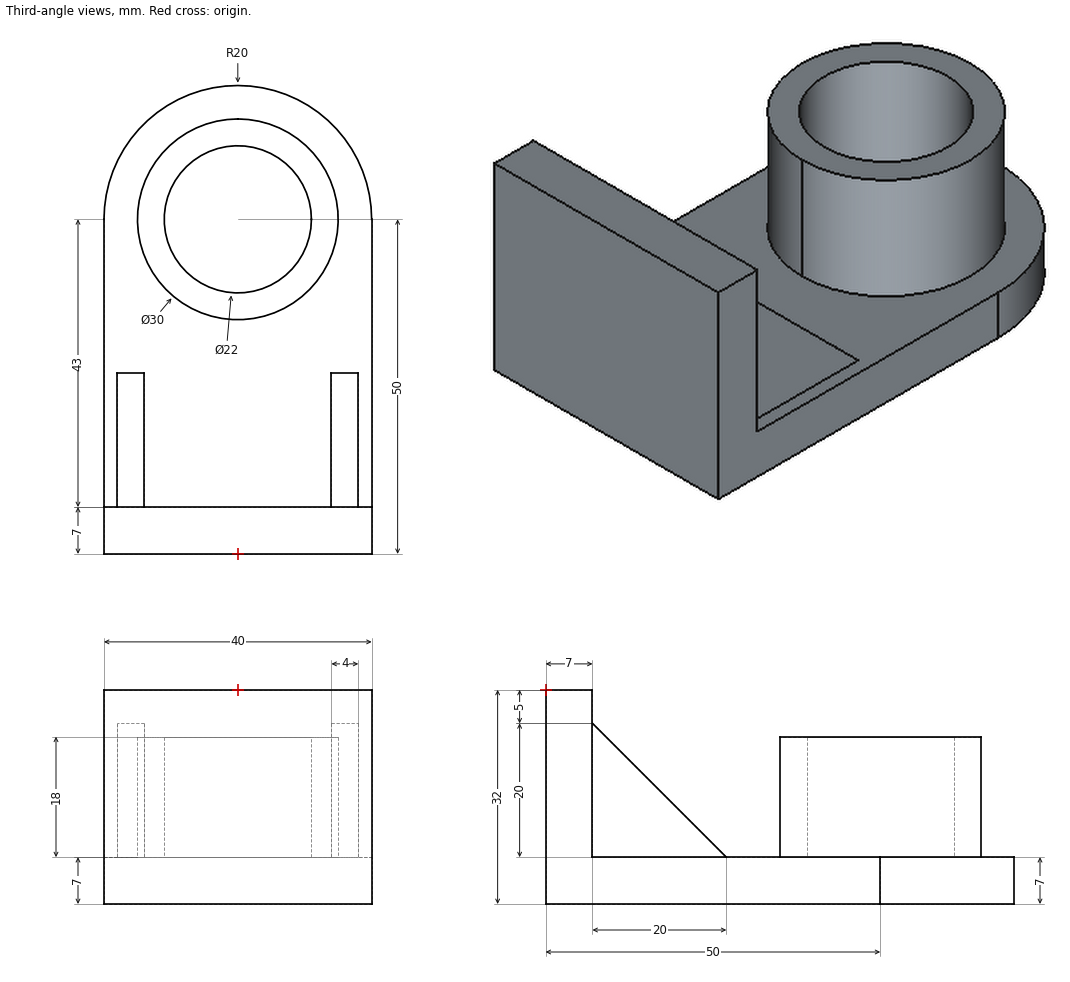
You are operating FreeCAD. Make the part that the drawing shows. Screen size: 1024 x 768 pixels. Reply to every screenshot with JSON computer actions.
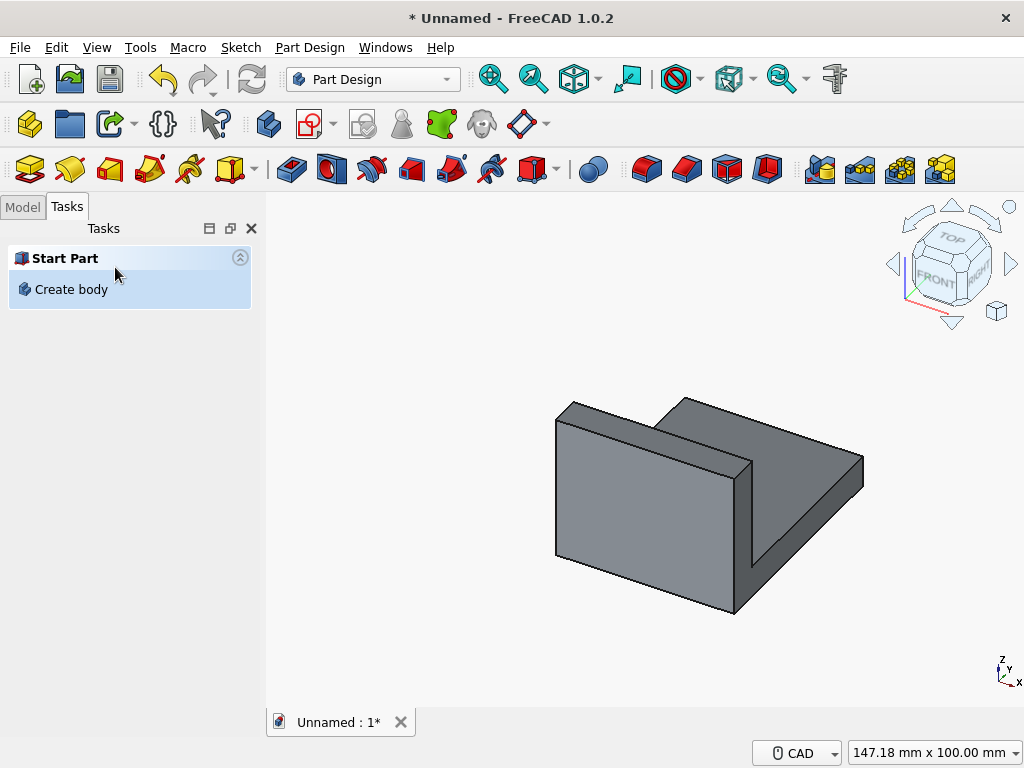
{"action": "key", "text": "0"}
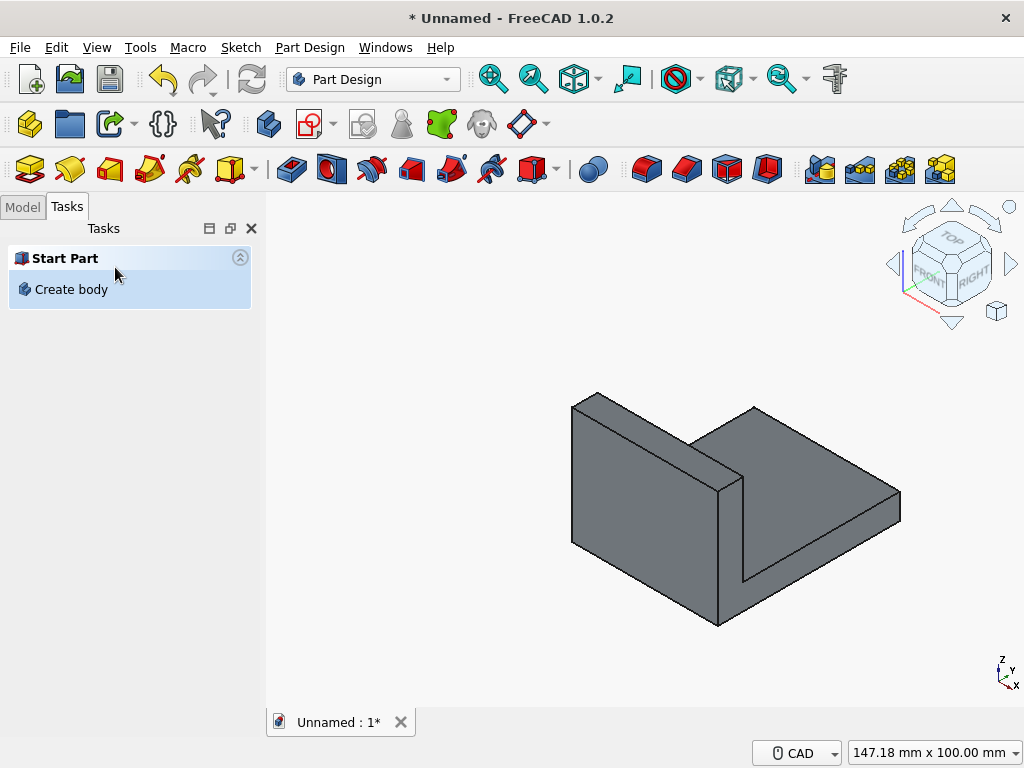
{"action": "left_click", "coordinate": [771, 481]}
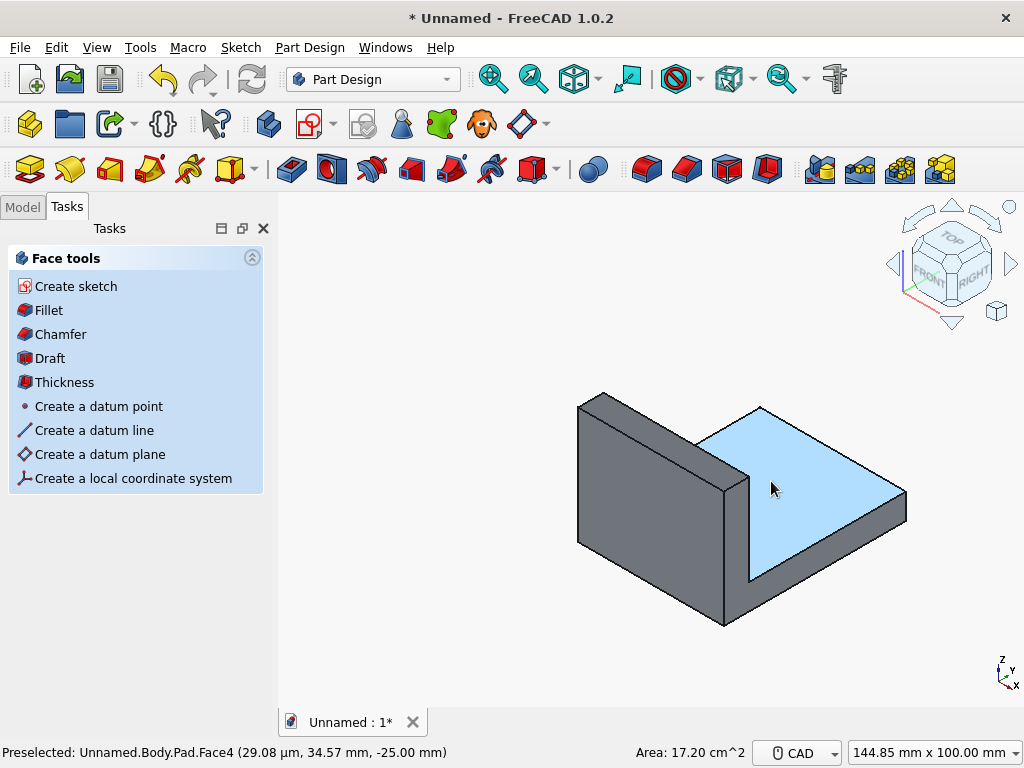
{"action": "left_click", "coordinate": [310, 124]}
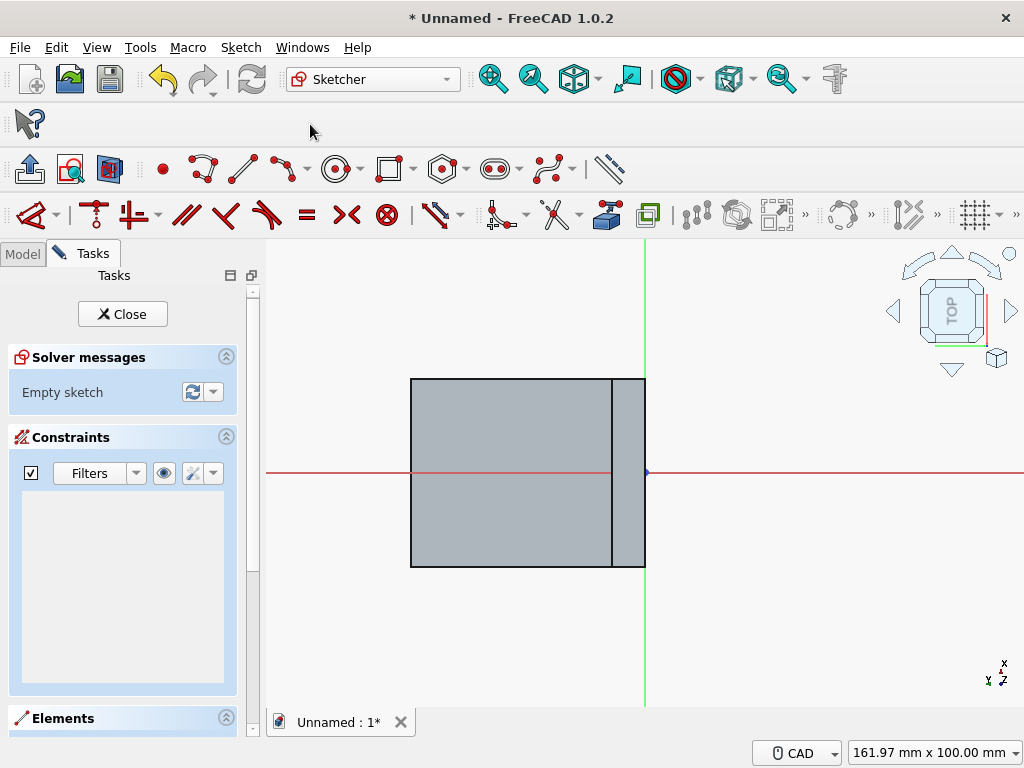
{"action": "scroll", "coordinate": [294, 473], "scroll_direction": "up", "scroll_amount": 1}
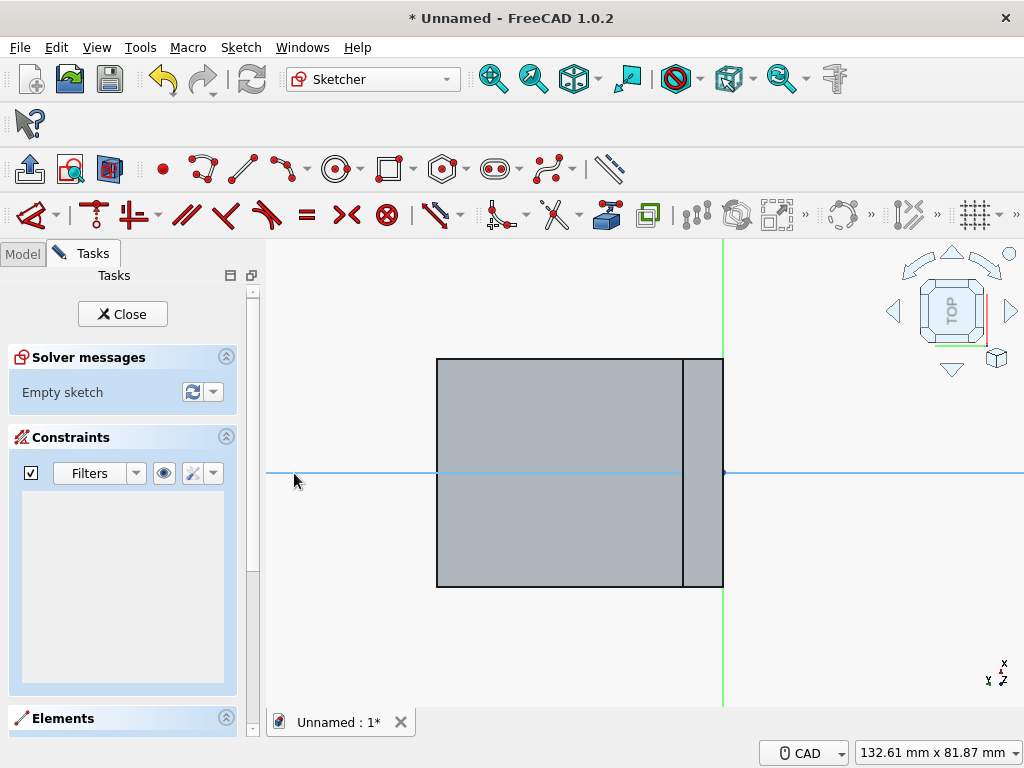
{"action": "key", "text": "g m"}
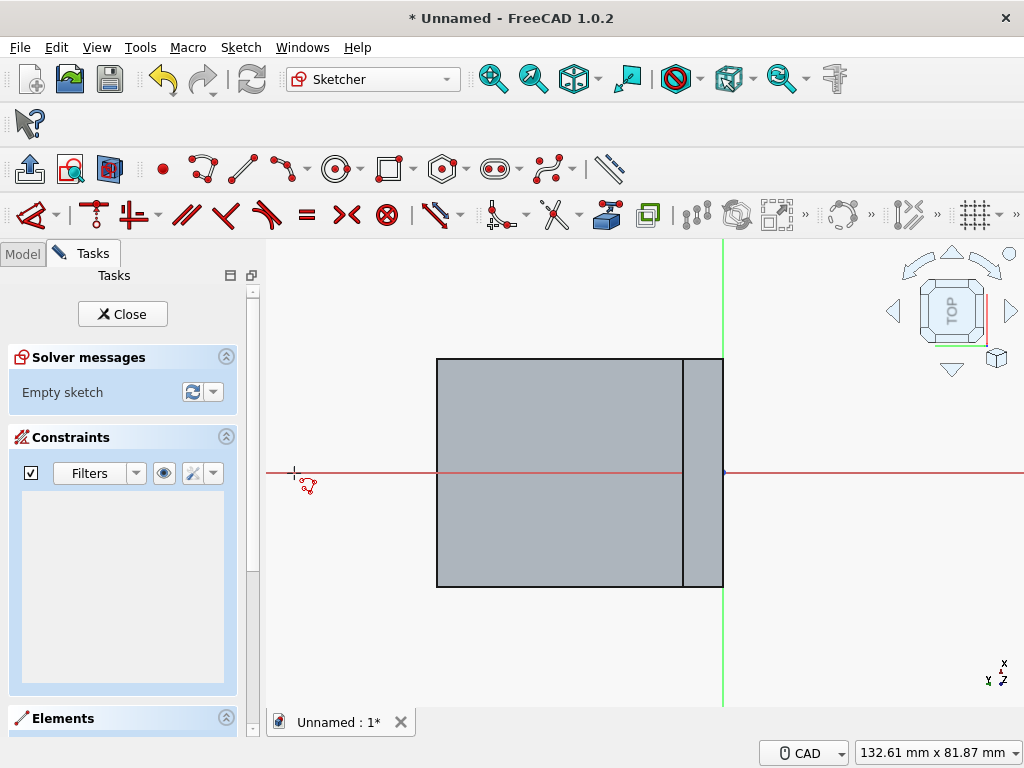
{"action": "left_click", "coordinate": [437, 587]}
{"action": "left_click", "coordinate": [683, 587]}
{"action": "left_click", "coordinate": [683, 359]}
{"action": "left_click", "coordinate": [437, 359]}
{"action": "right_click", "coordinate": [437, 359]}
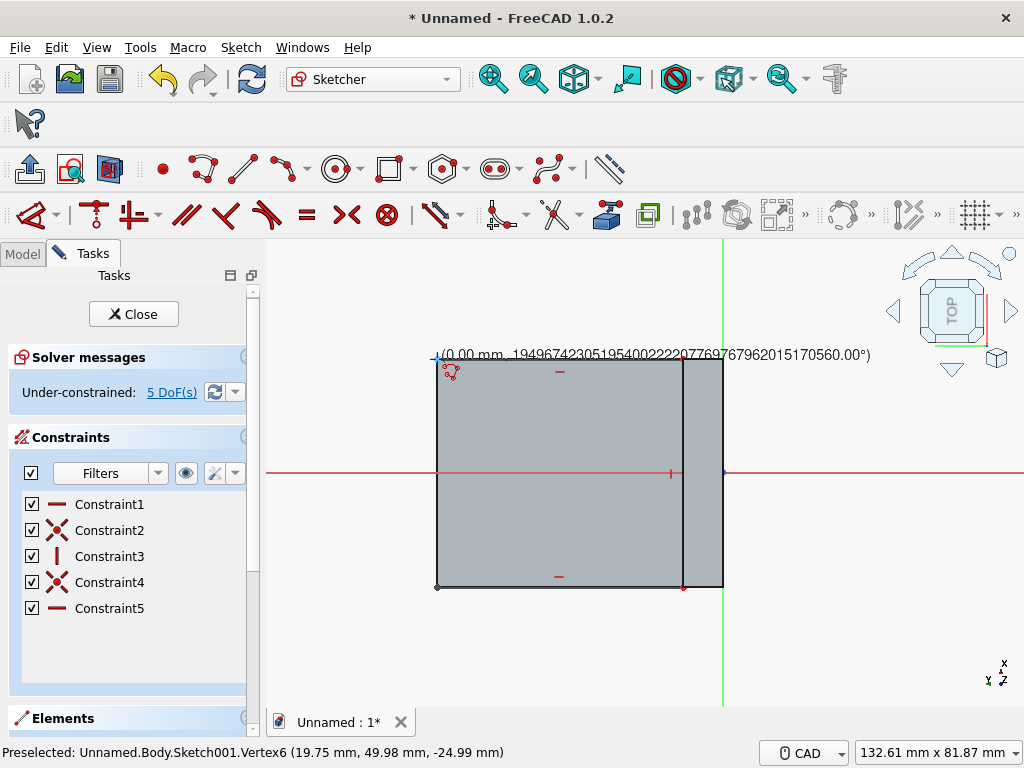
{"action": "left_click", "coordinate": [284, 170]}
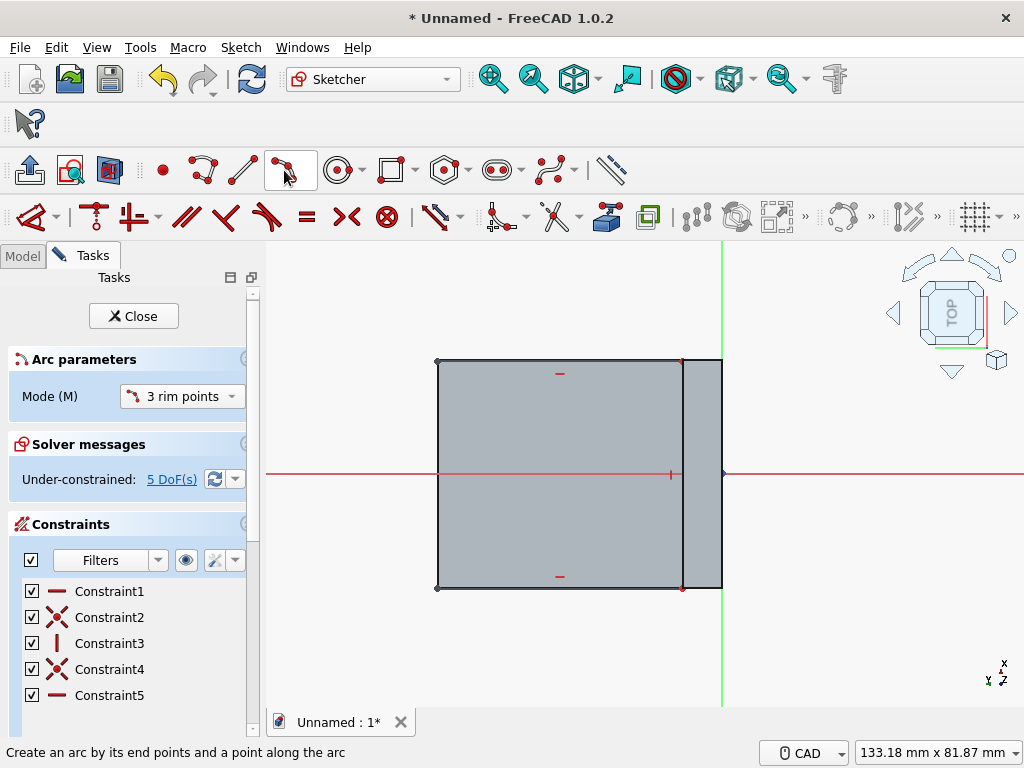
{"action": "left_click", "coordinate": [438, 361]}
{"action": "left_click", "coordinate": [438, 589]}
{"action": "left_click", "coordinate": [330, 439]}
{"action": "key", "text": "Escape"}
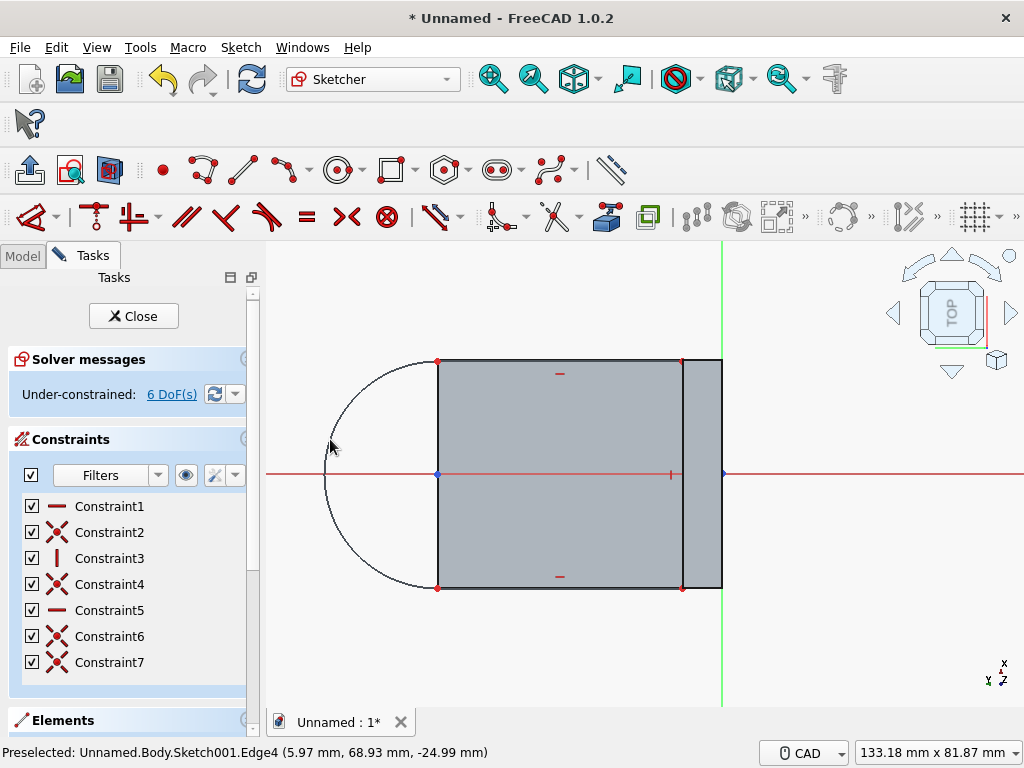
{"action": "left_click", "coordinate": [511, 589]}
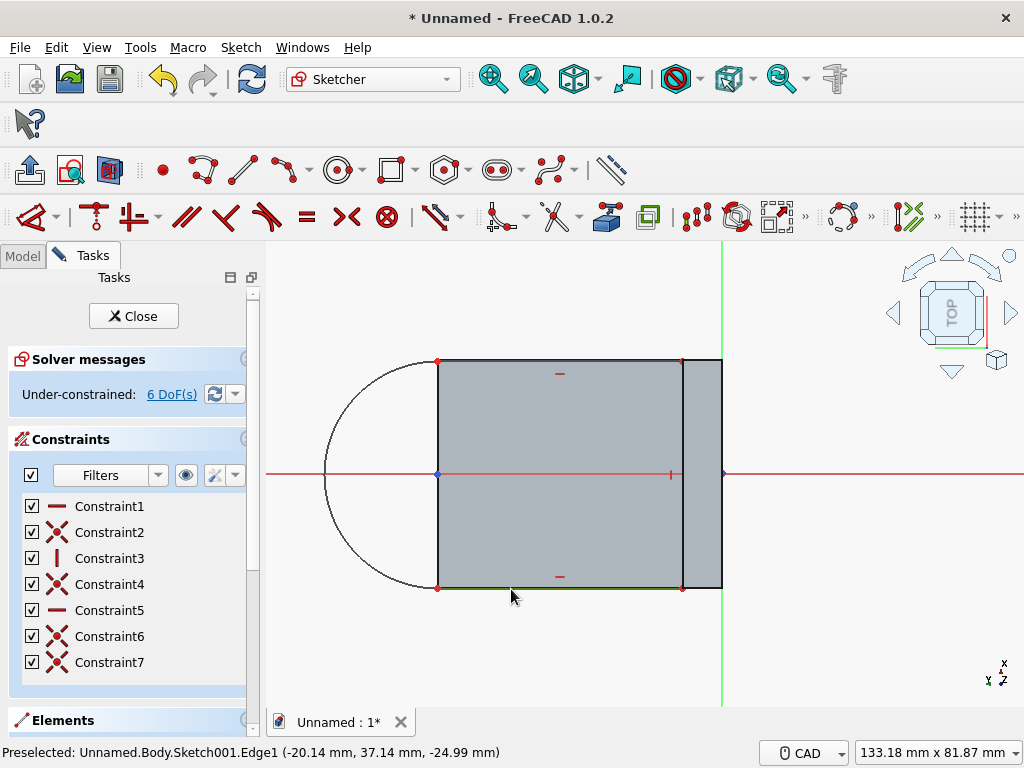
{"action": "left_click", "coordinate": [346, 408]}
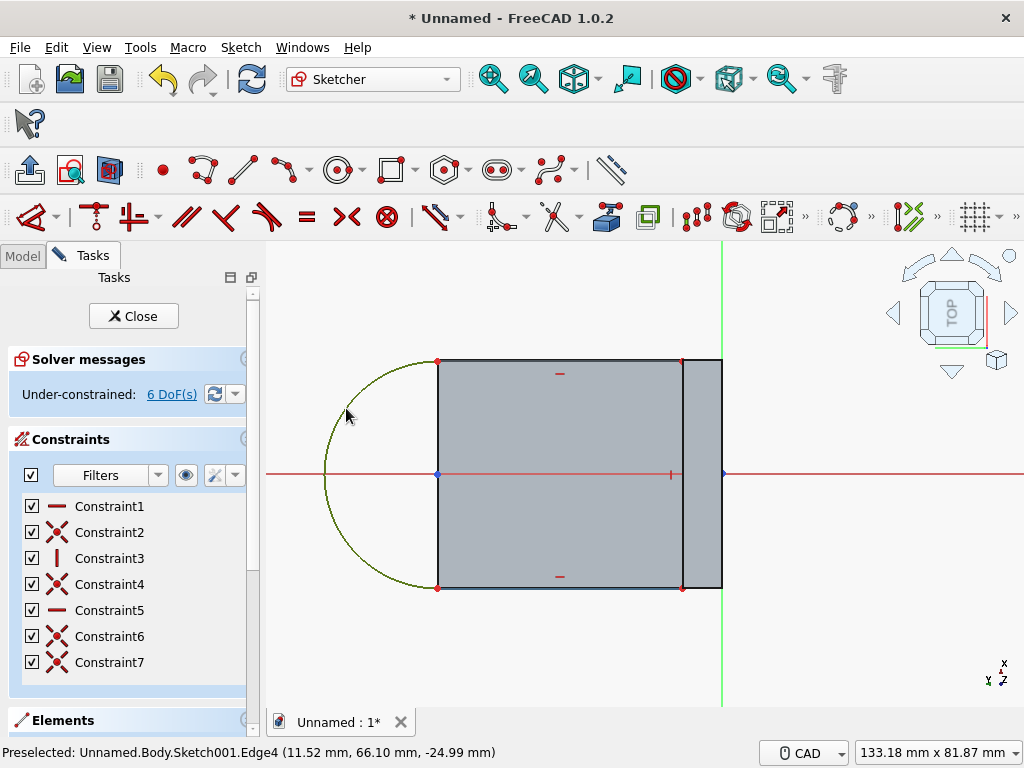
{"action": "left_click", "coordinate": [268, 218]}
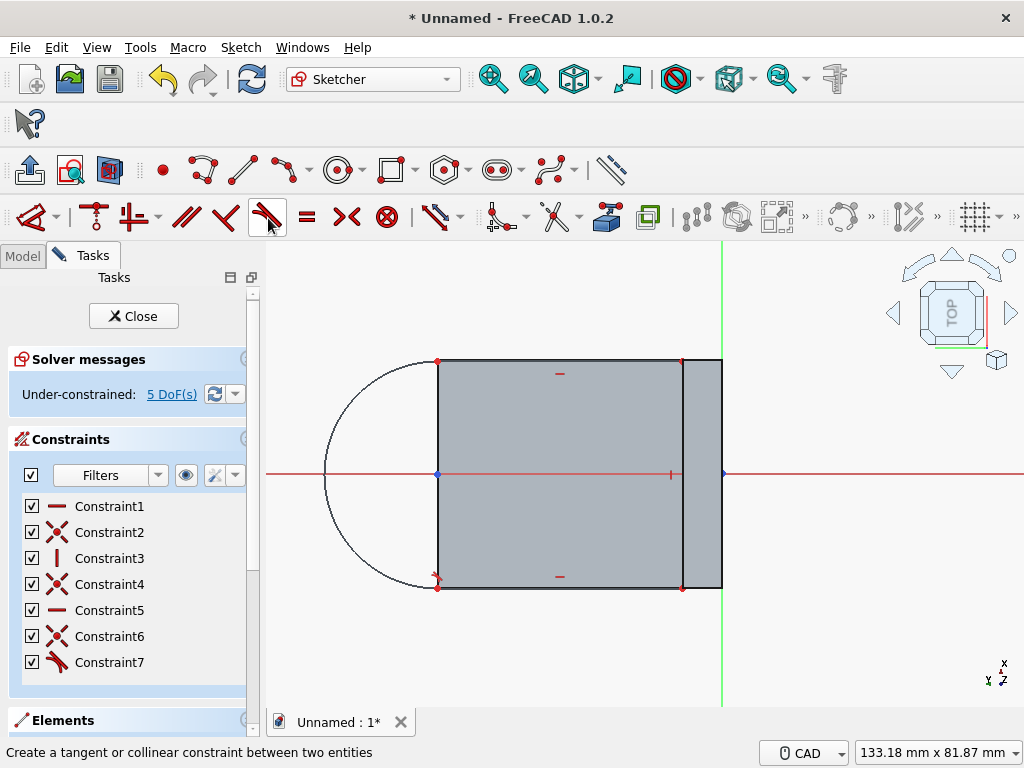
{"action": "left_click", "coordinate": [609, 361]}